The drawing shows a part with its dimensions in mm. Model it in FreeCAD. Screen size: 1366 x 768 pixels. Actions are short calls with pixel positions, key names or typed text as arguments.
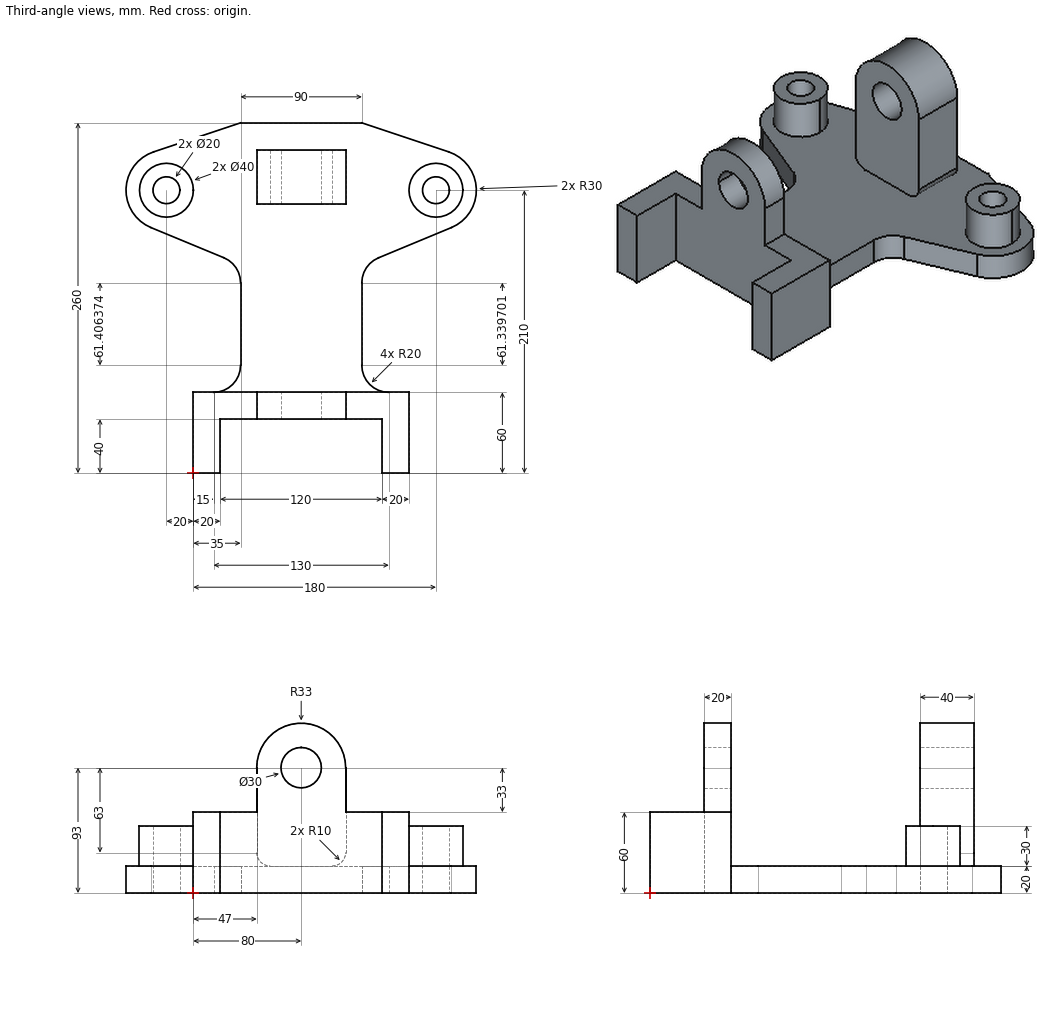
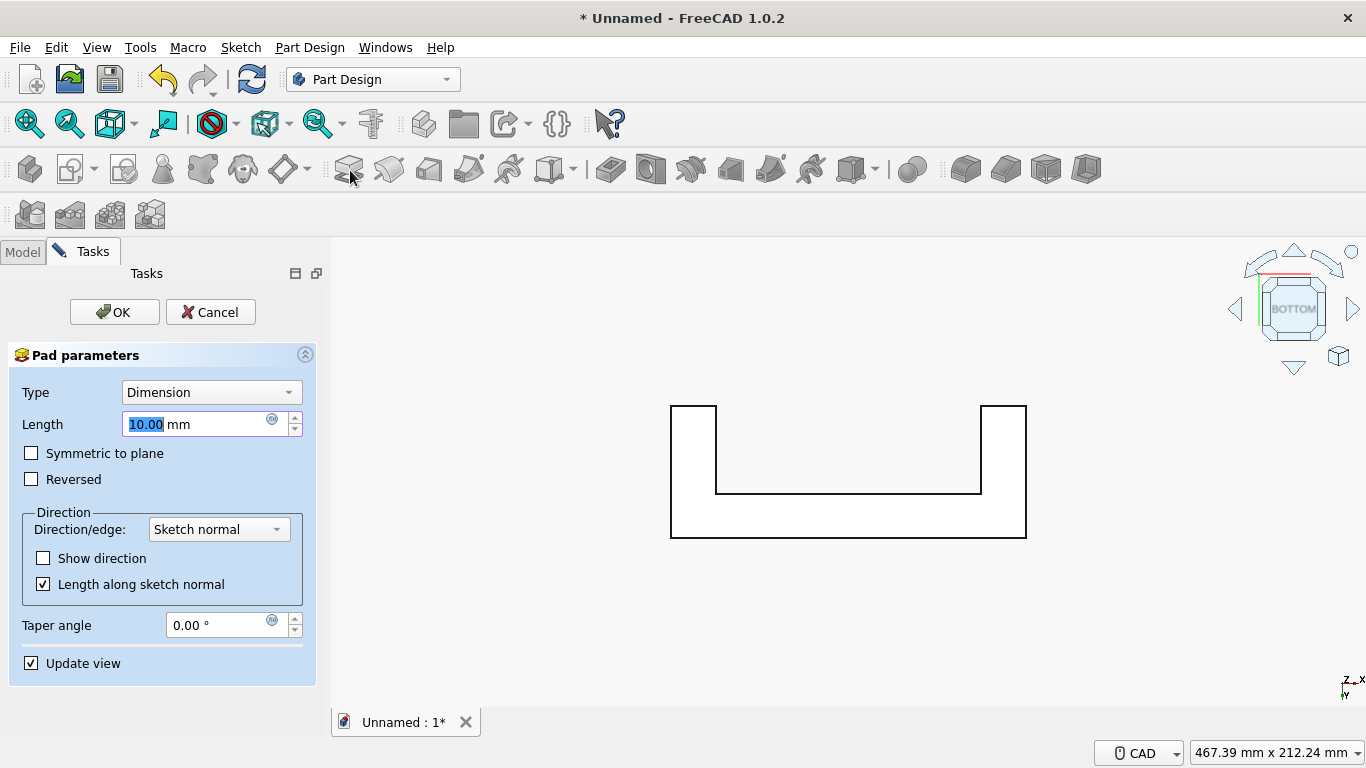
text(20)
key(Tab)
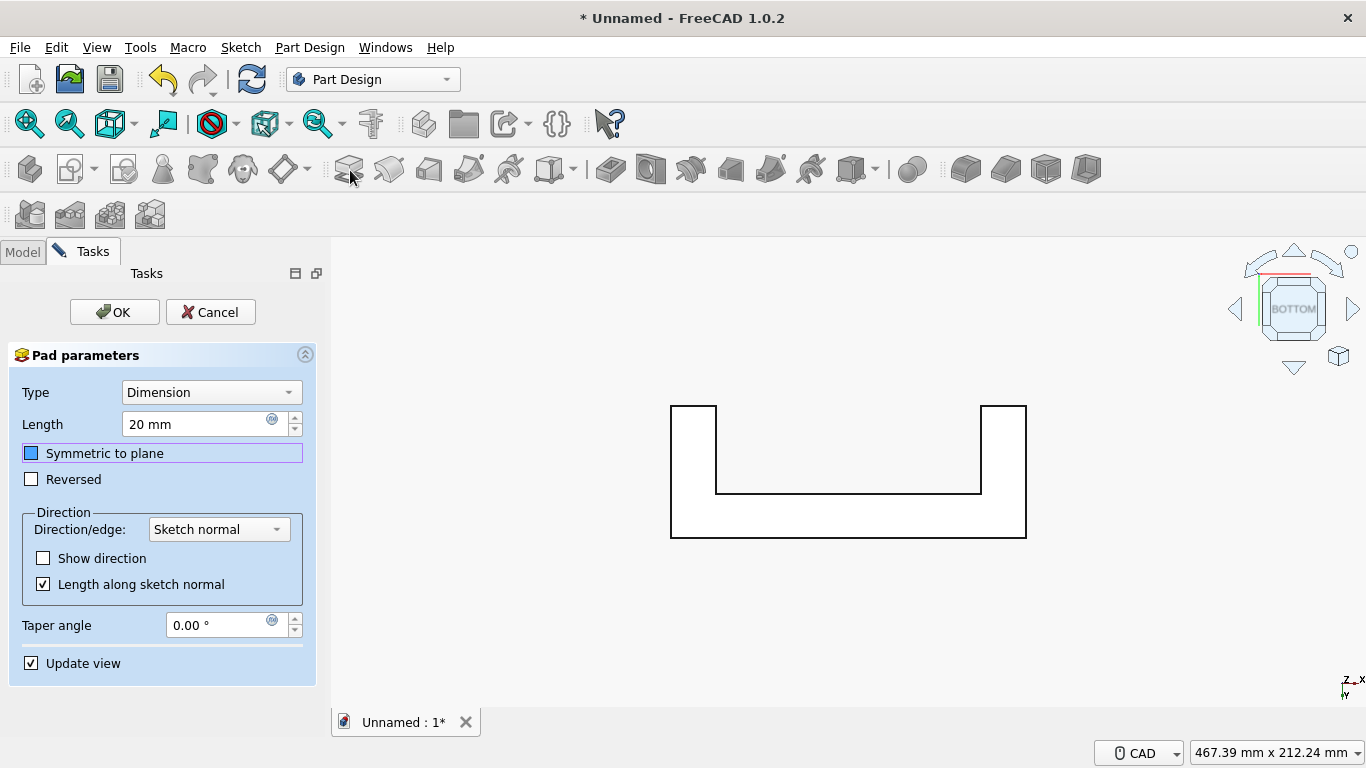
click(30, 479)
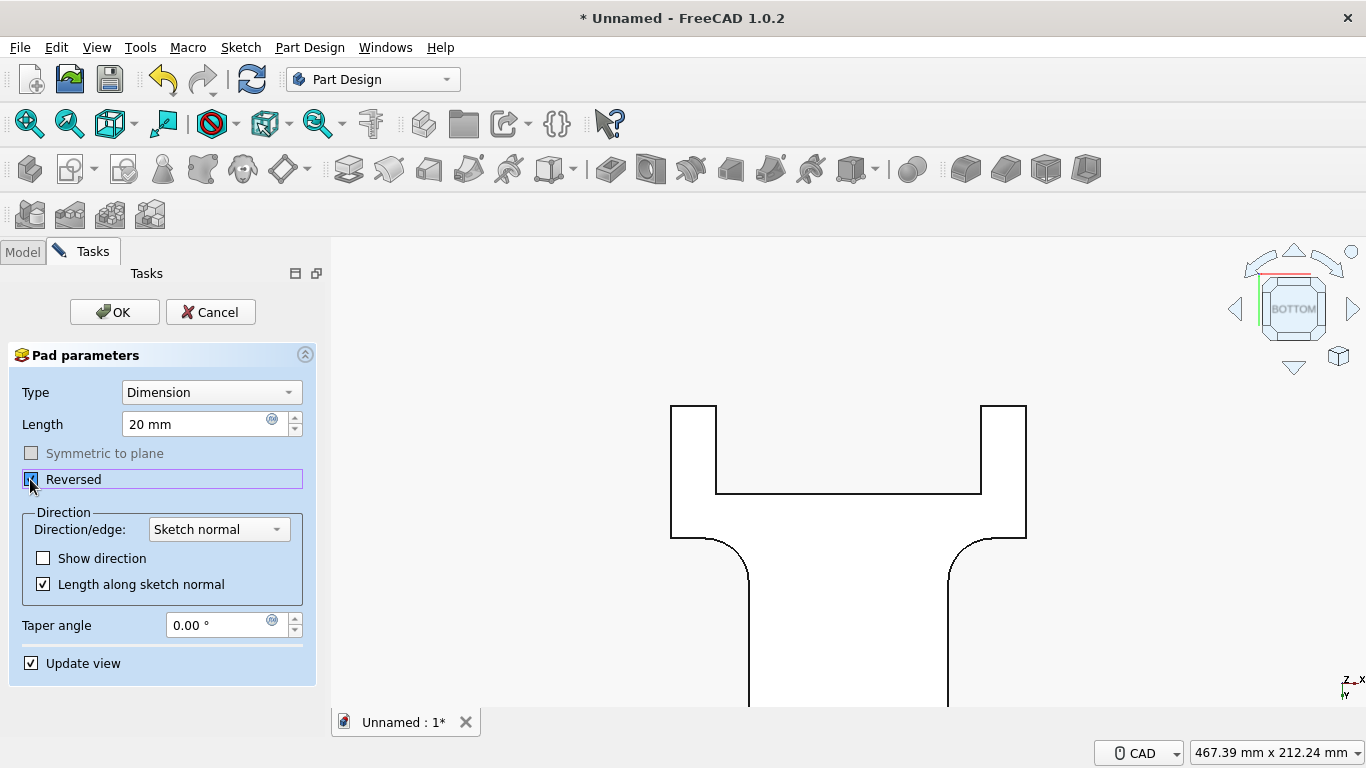
click(115, 312)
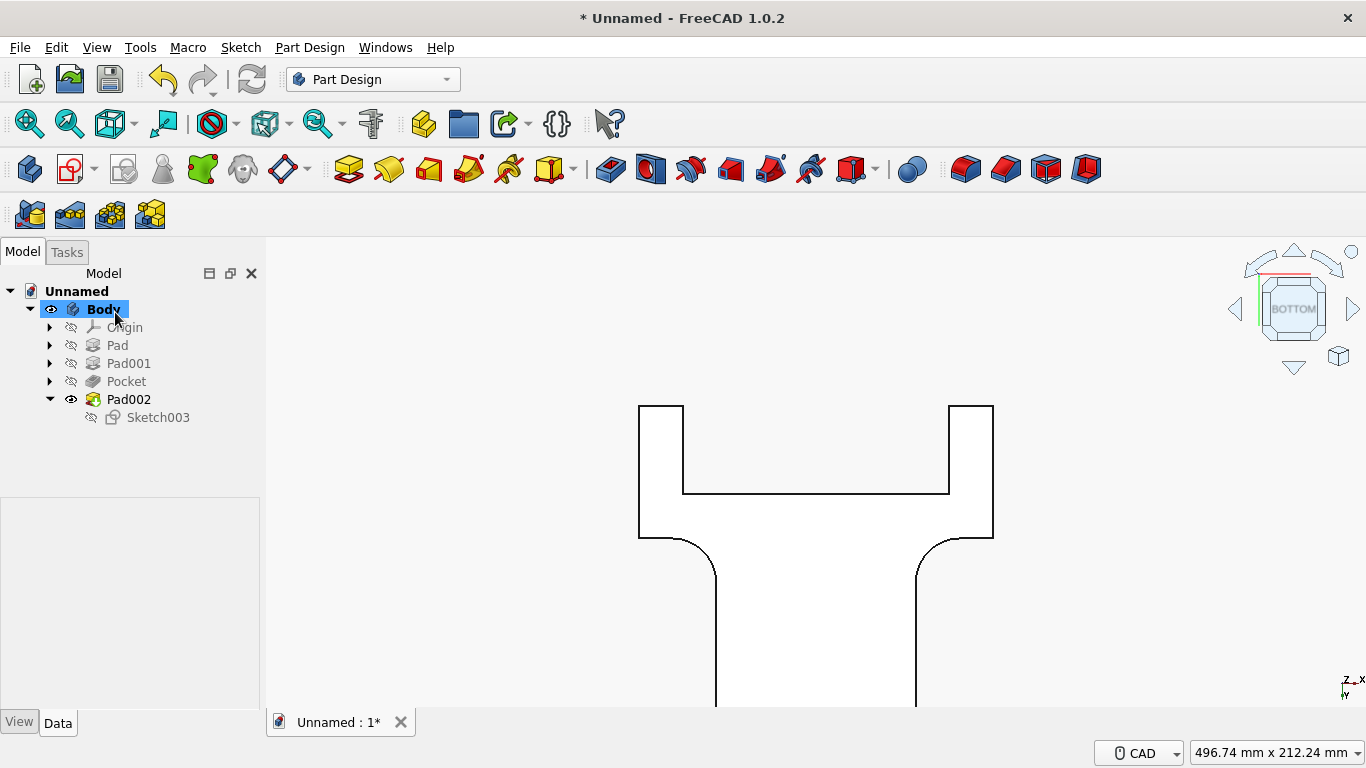
click(30, 124)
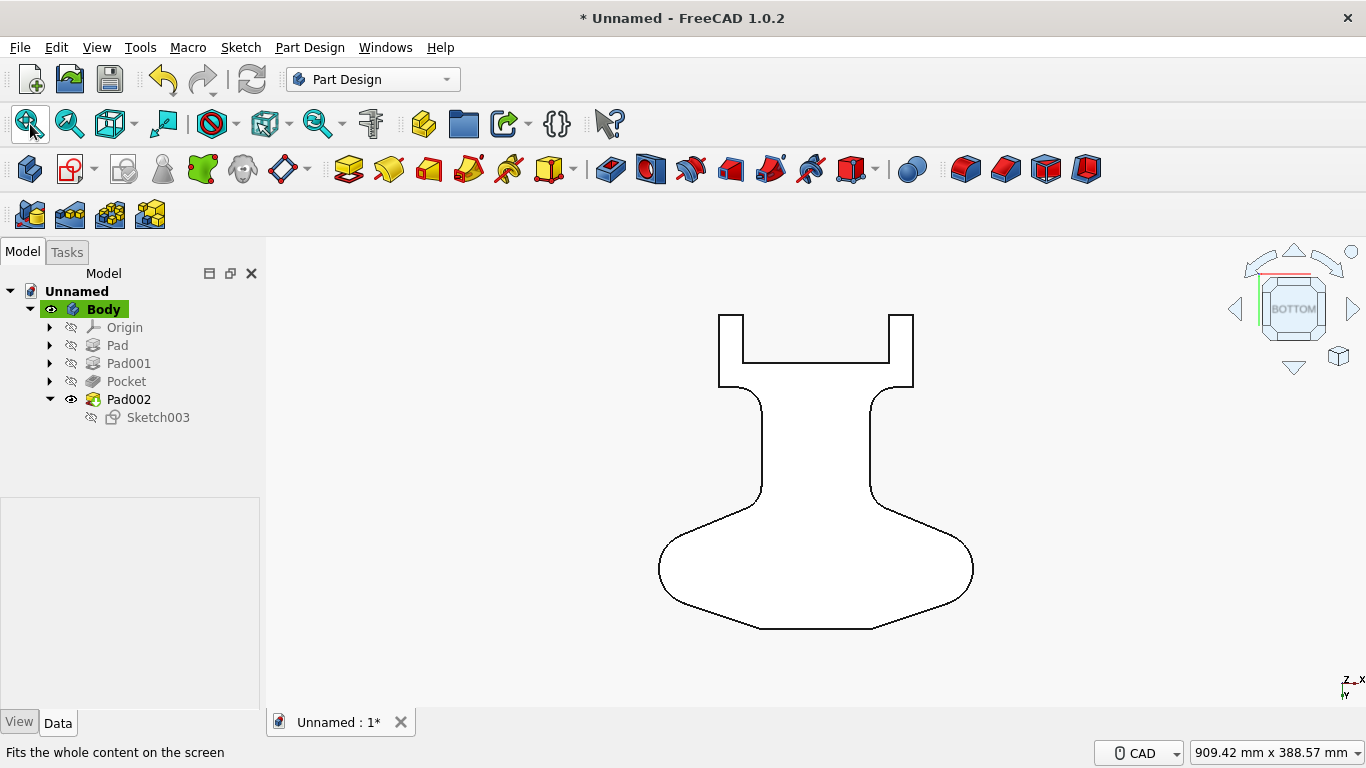
key(0)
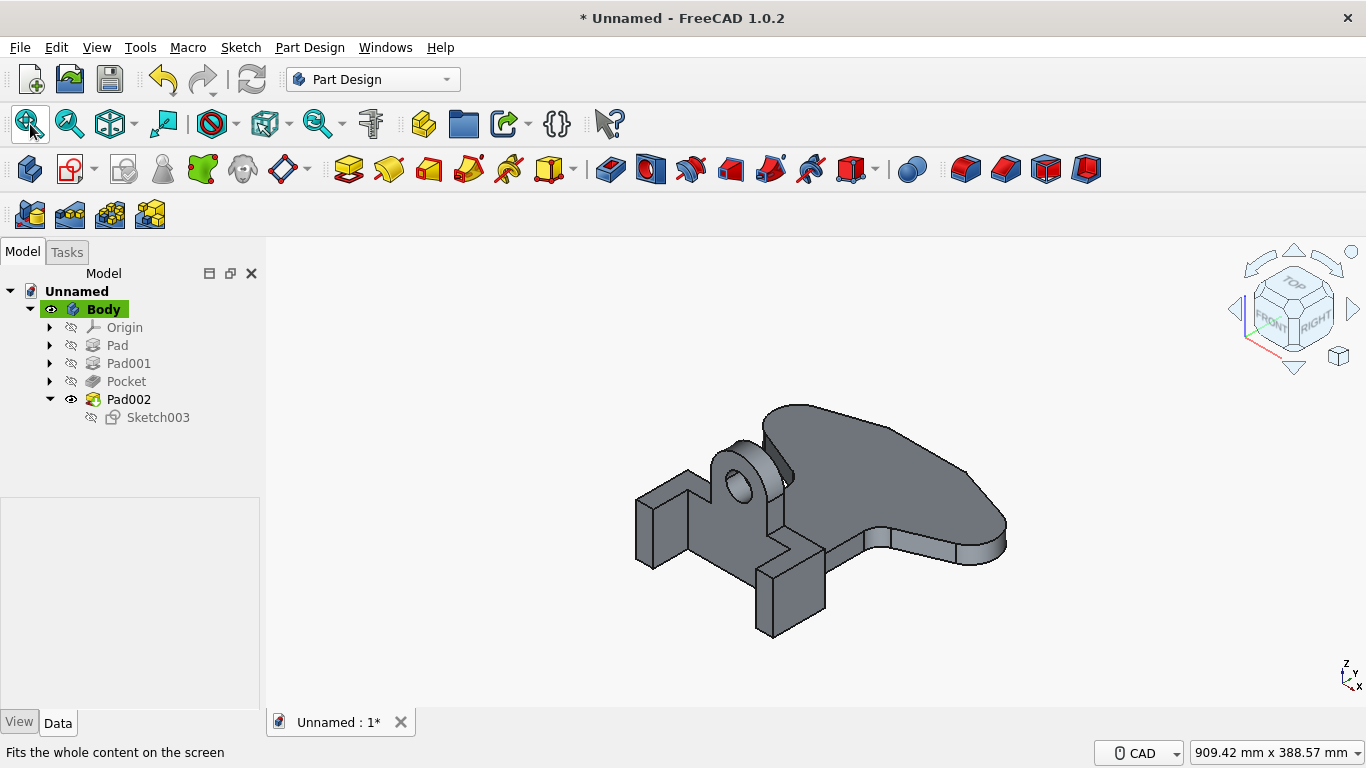
click(866, 485)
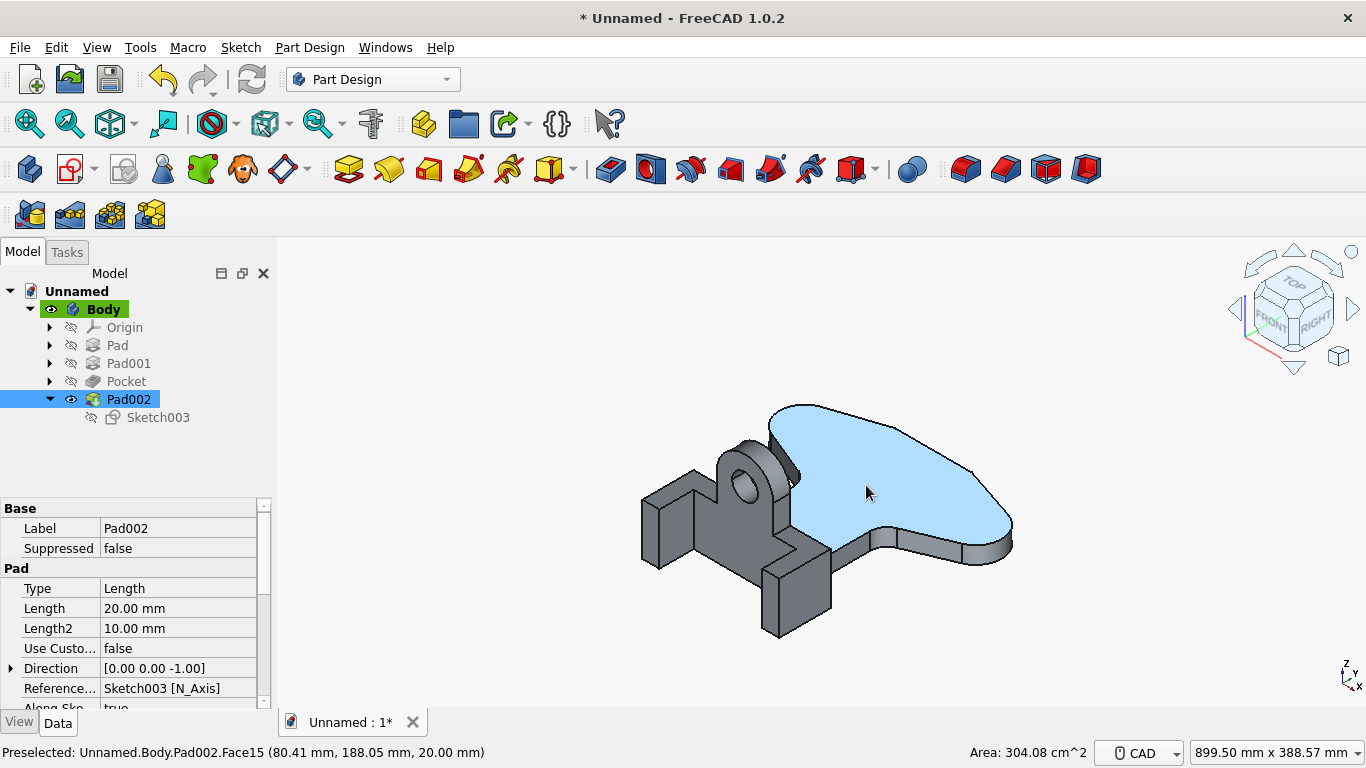
click(70, 170)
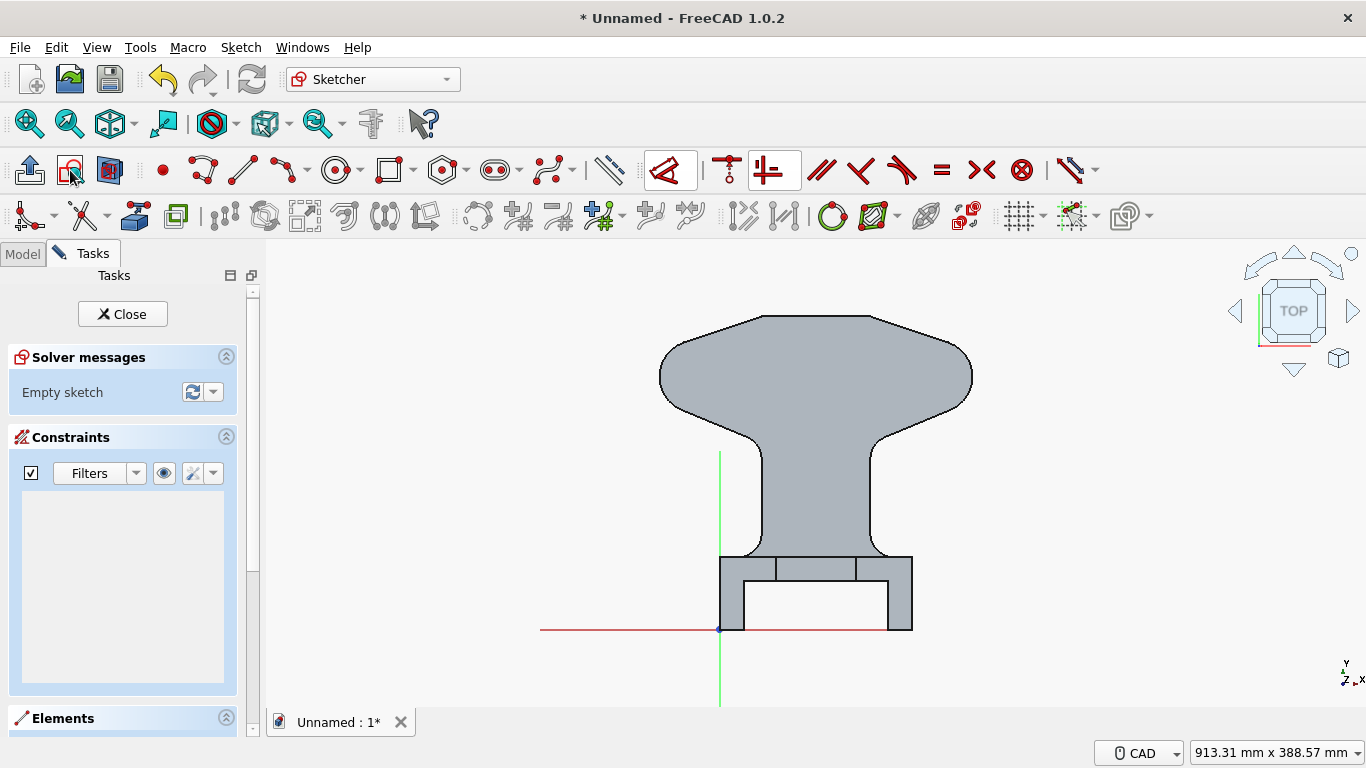
key(q)
key(s)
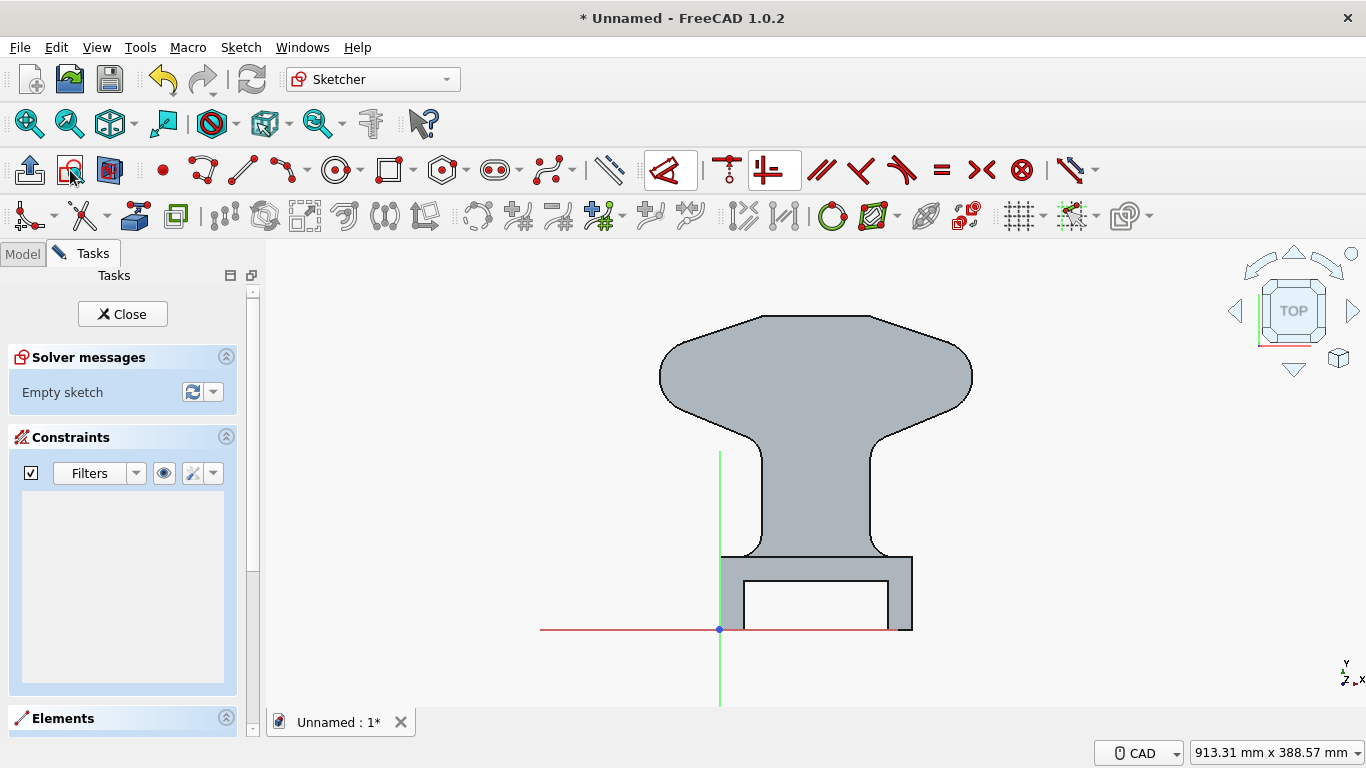
click(336, 170)